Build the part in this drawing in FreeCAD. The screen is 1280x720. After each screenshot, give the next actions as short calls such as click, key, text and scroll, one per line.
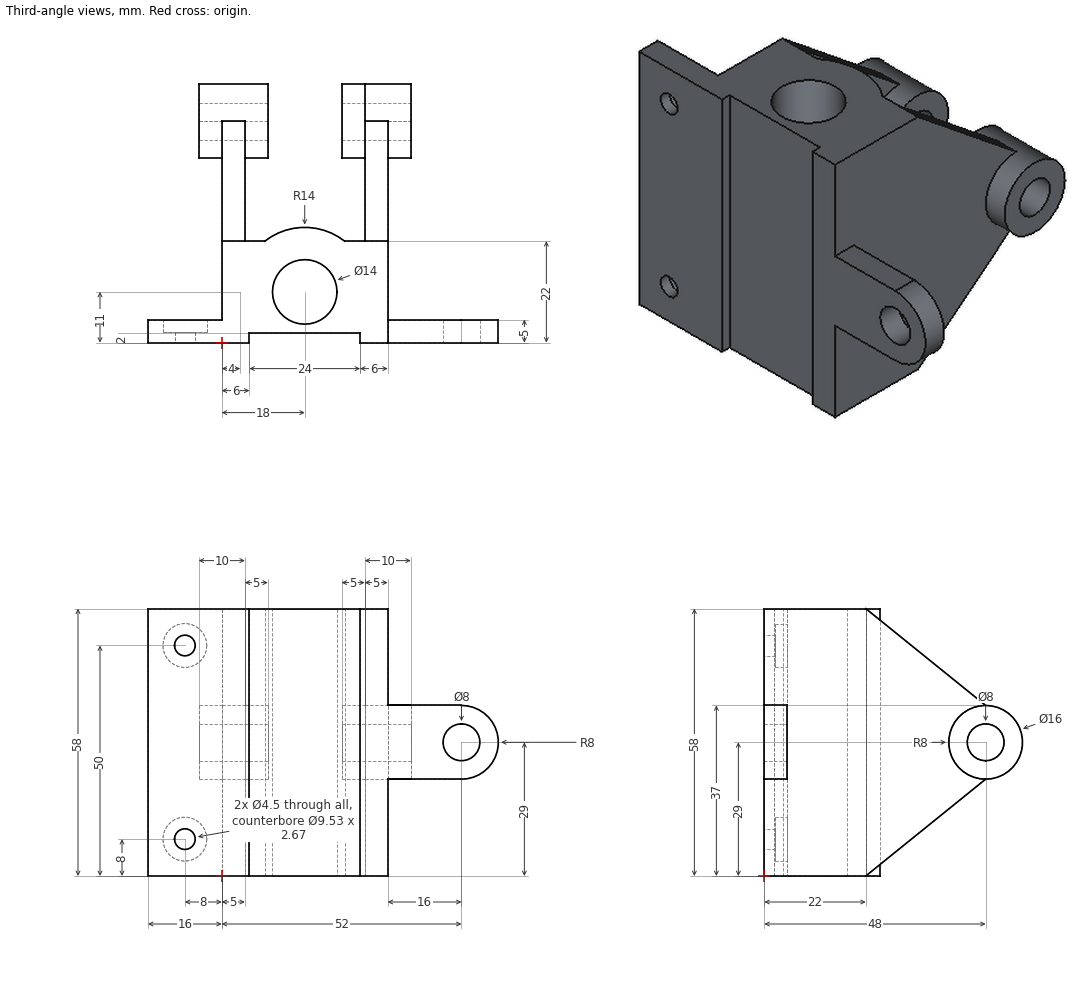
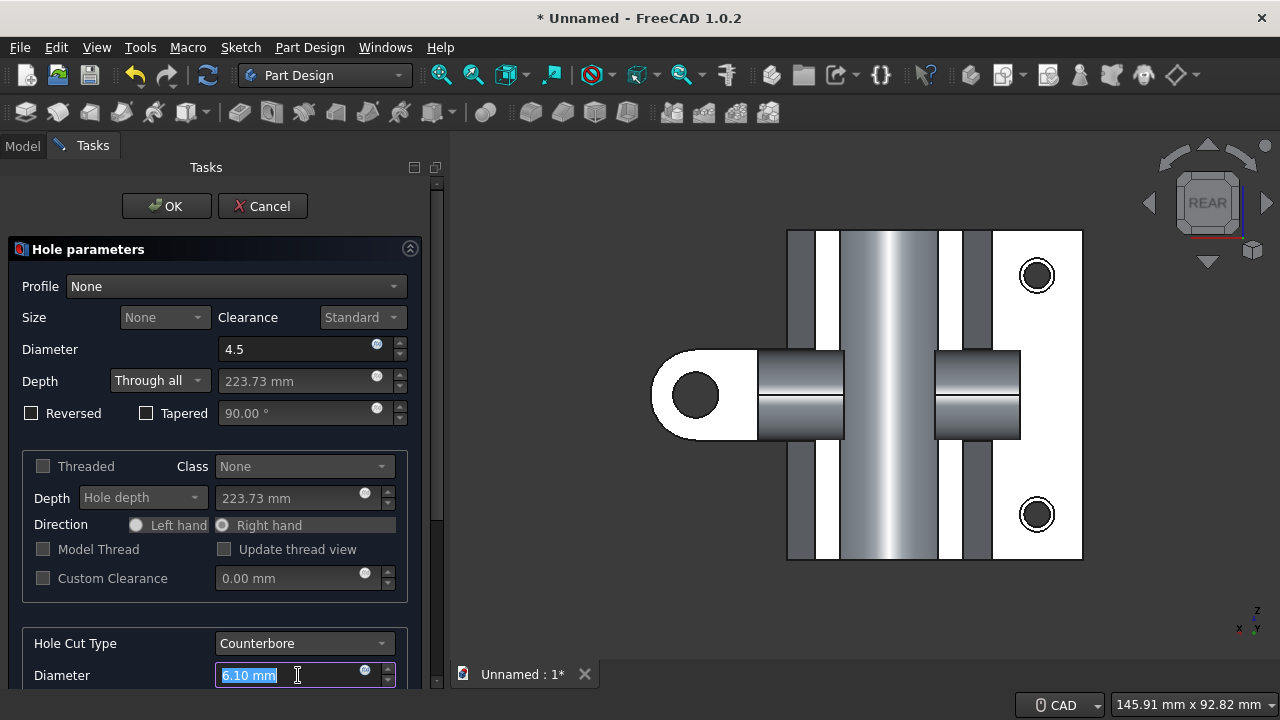
text(9.53)
key(Tab)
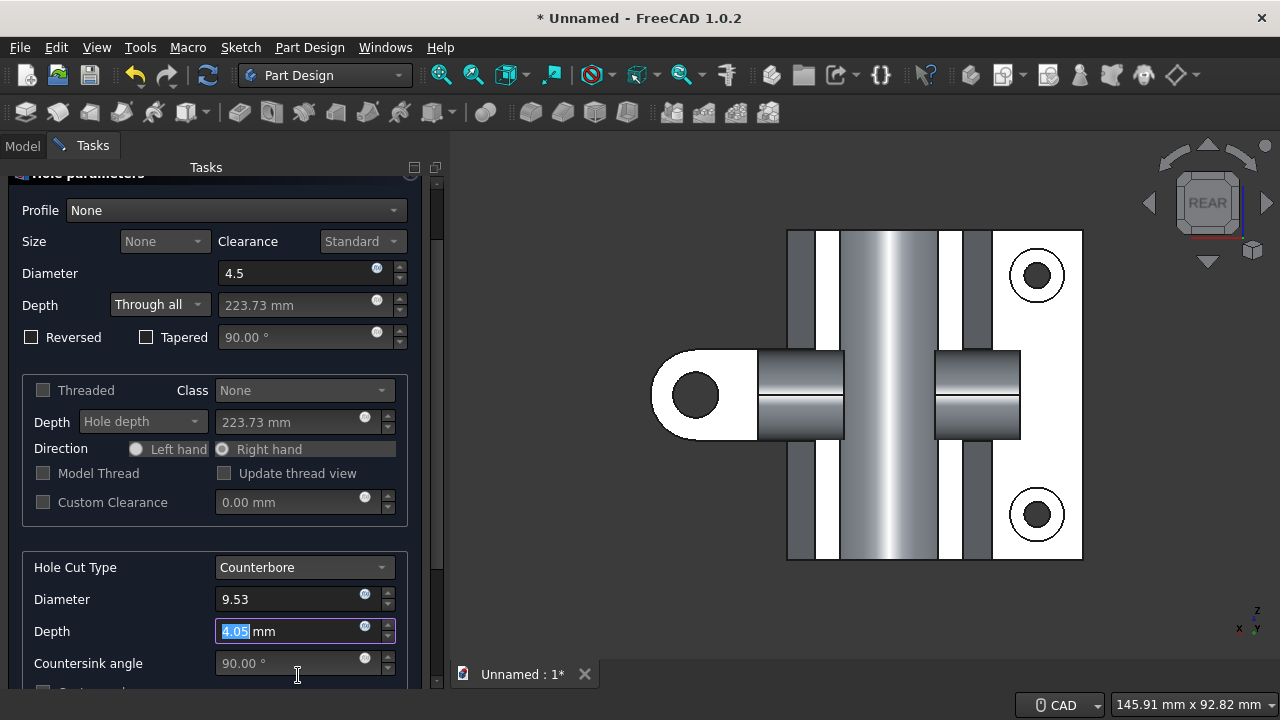
text(2.67)
key(Tab)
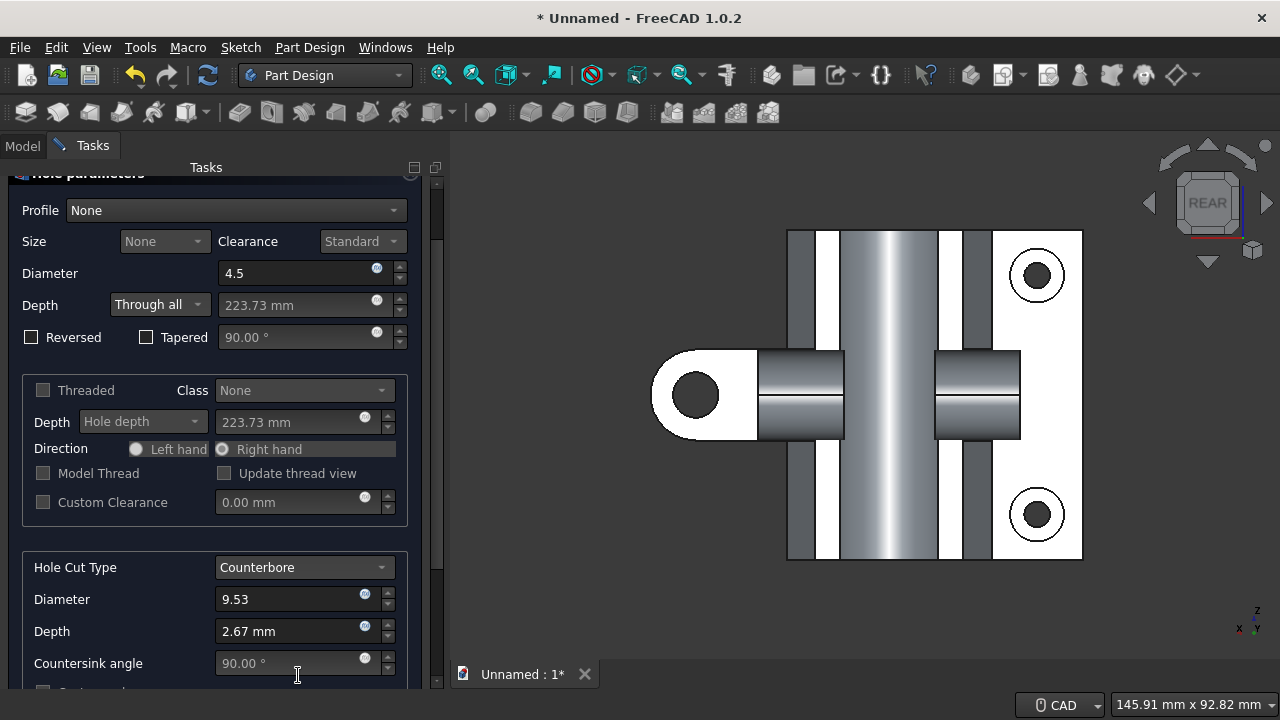
scroll(437, 432, up, 3)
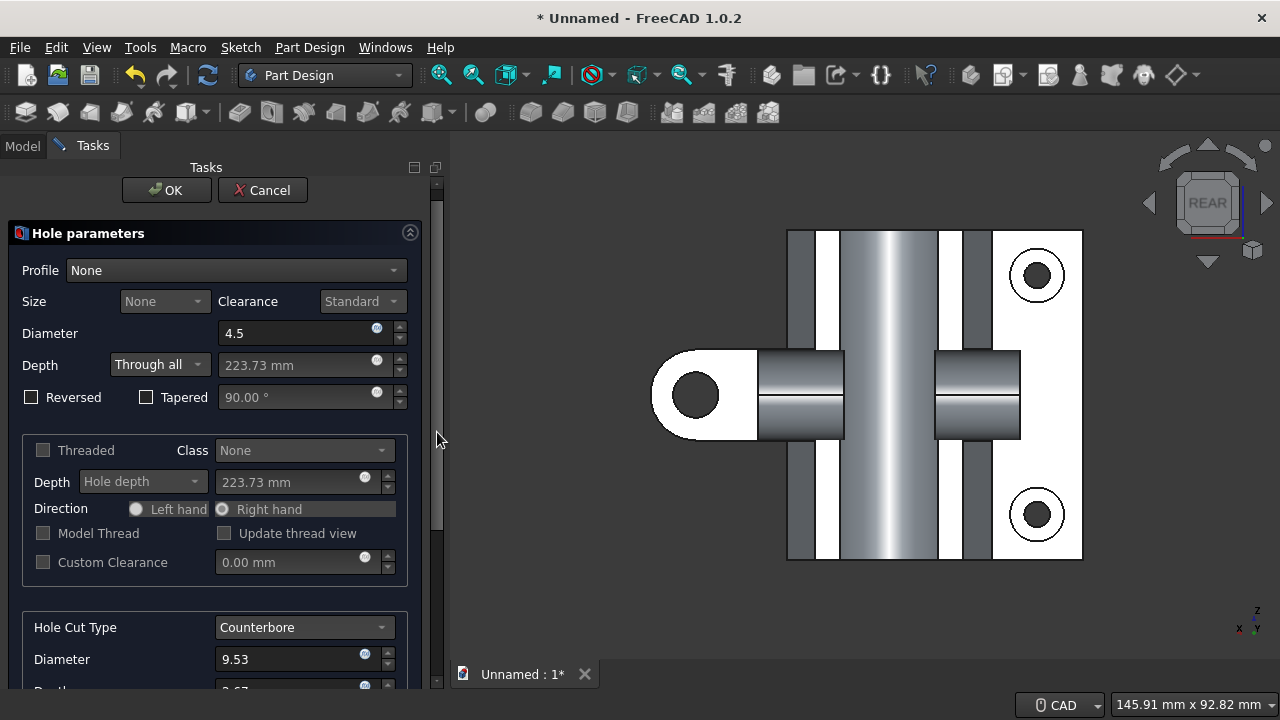
click(167, 206)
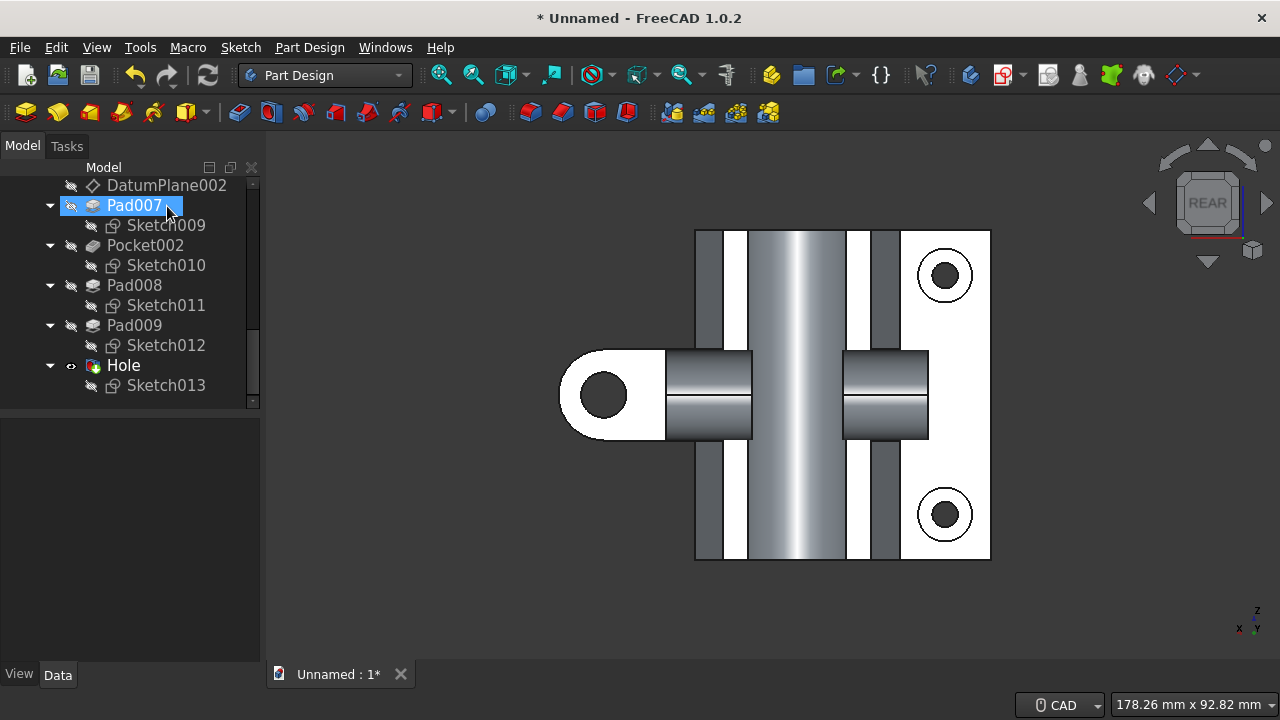
key(0)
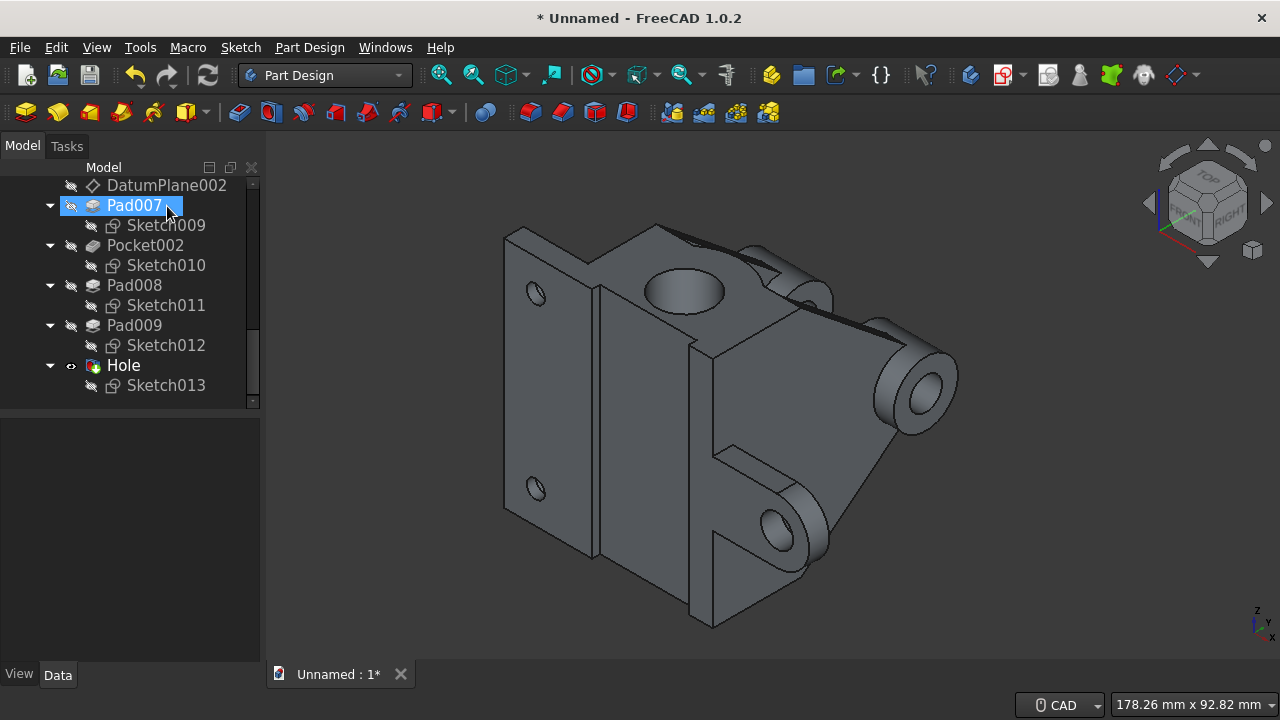
key(v)
key(f)